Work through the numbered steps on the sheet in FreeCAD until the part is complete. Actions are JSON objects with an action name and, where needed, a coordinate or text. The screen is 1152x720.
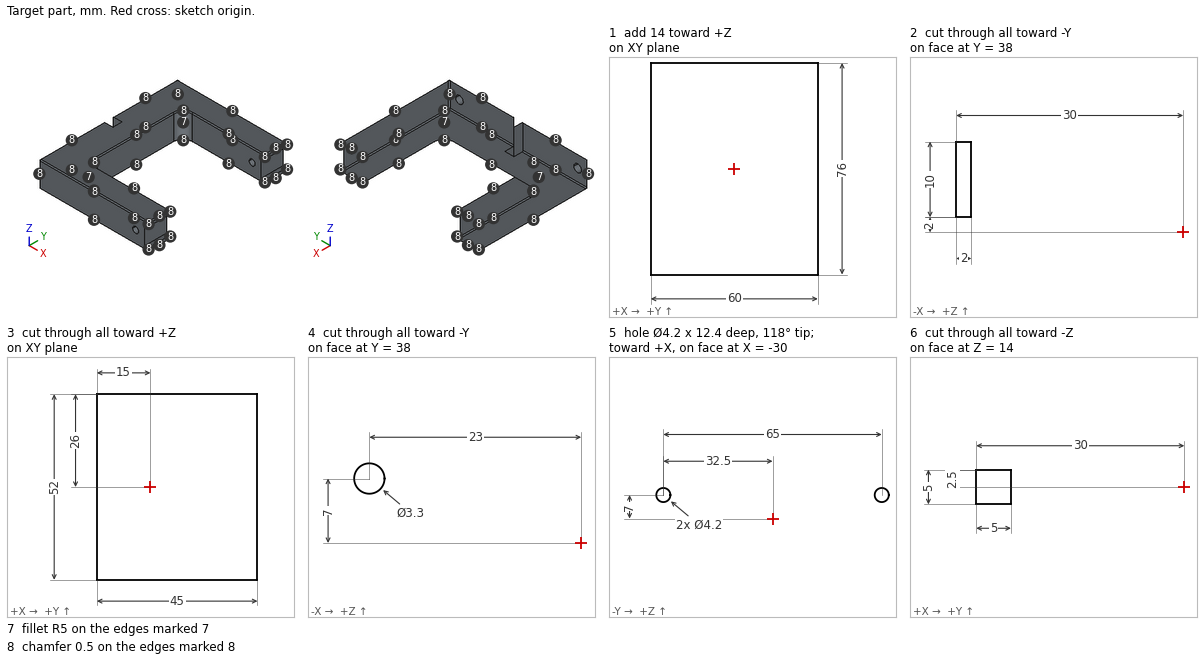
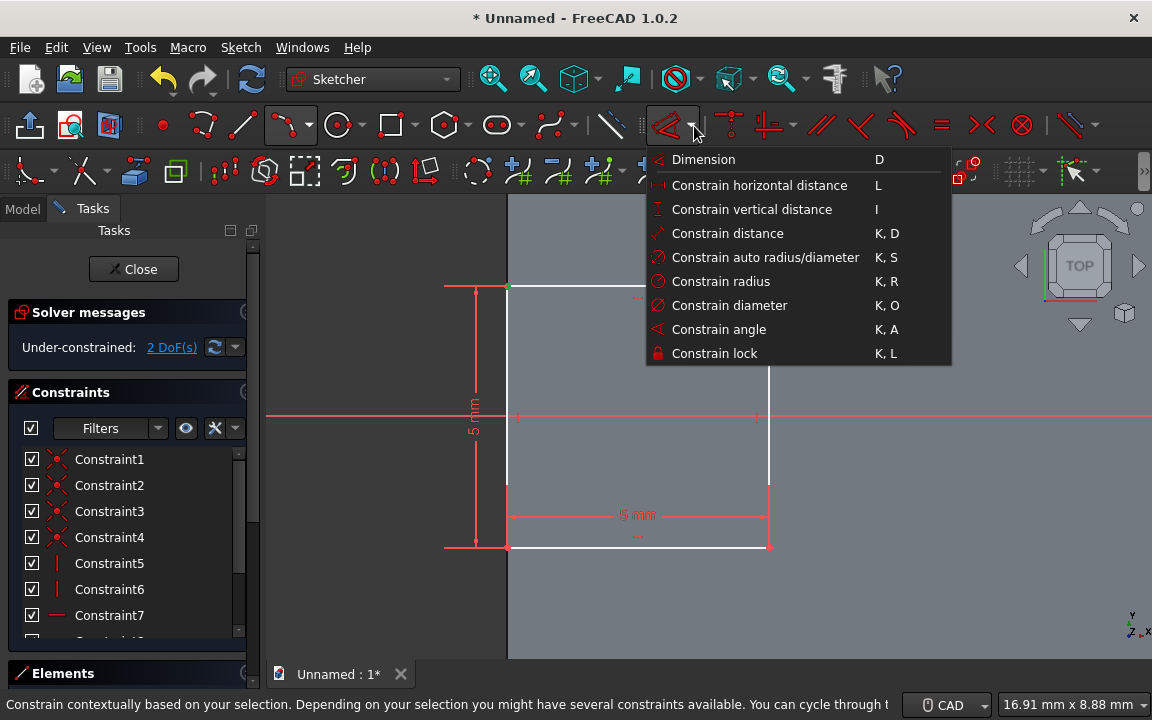
{"action": "left_click", "coordinate": [799, 185]}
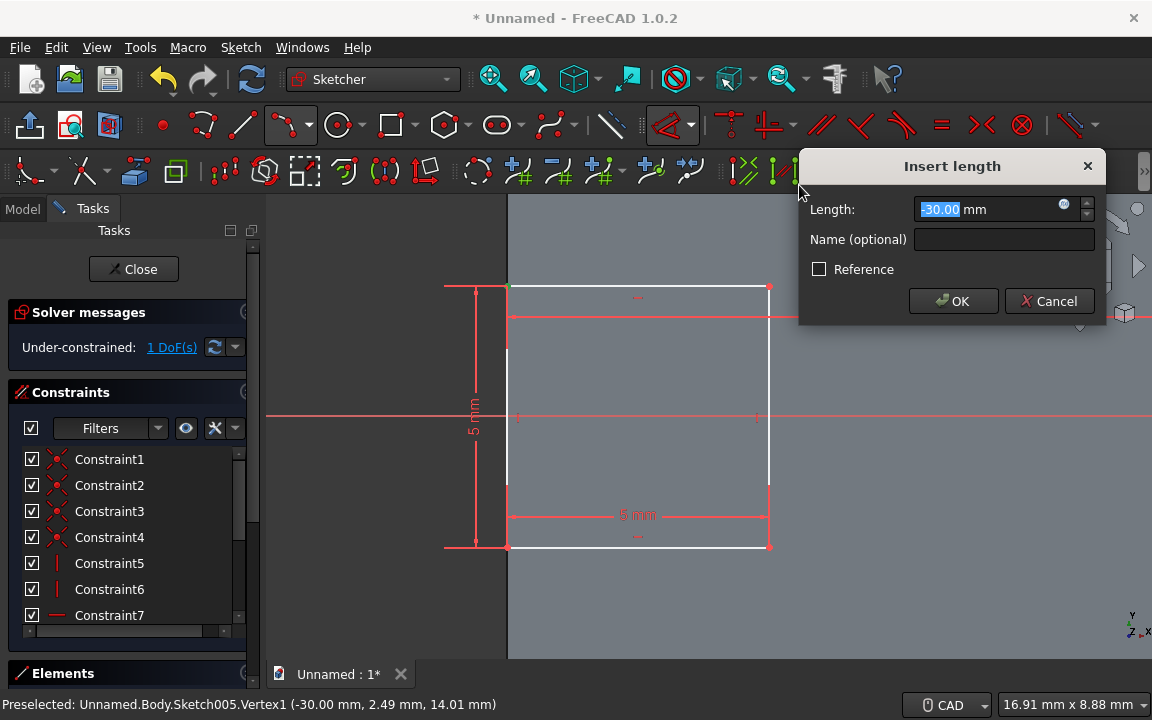
{"action": "type", "text": "-30"}
{"action": "key", "text": "Return"}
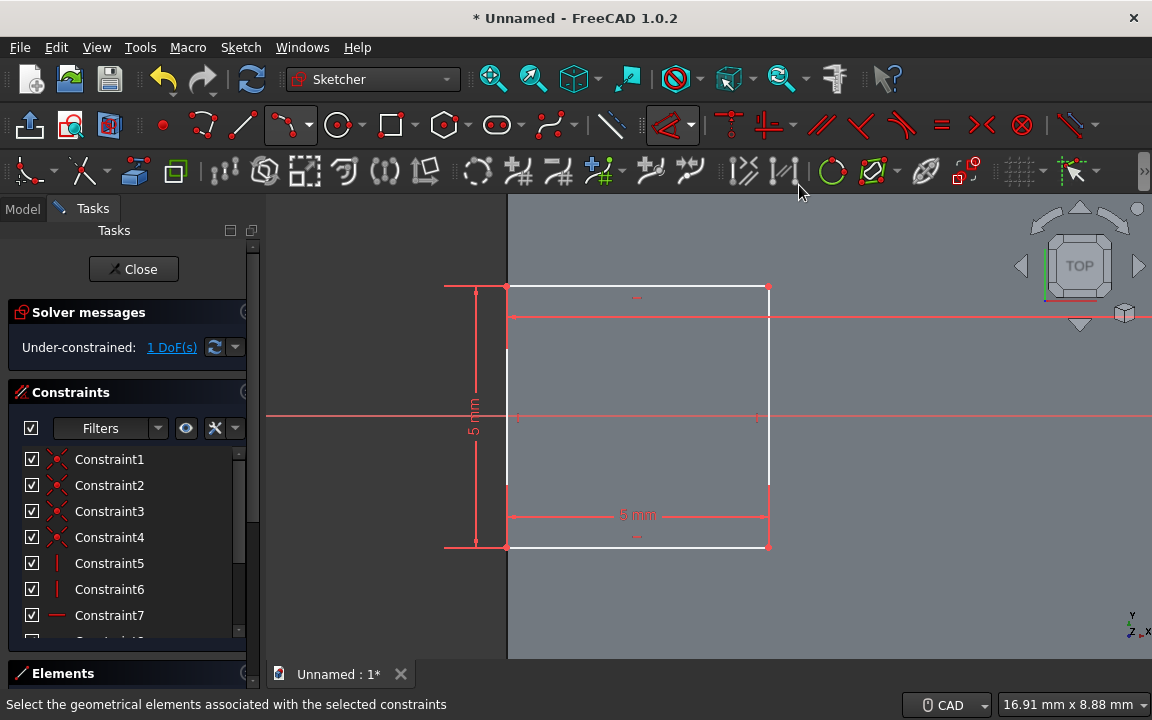
{"action": "left_click", "coordinate": [507, 286]}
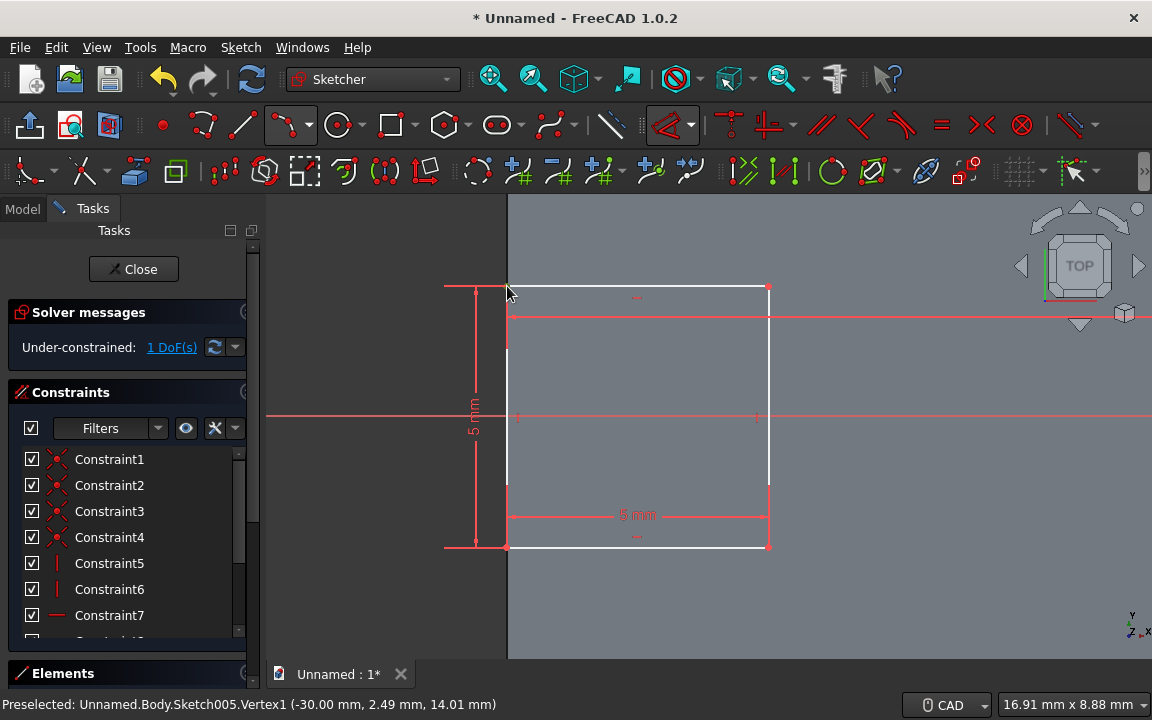
{"action": "key", "text": "i"}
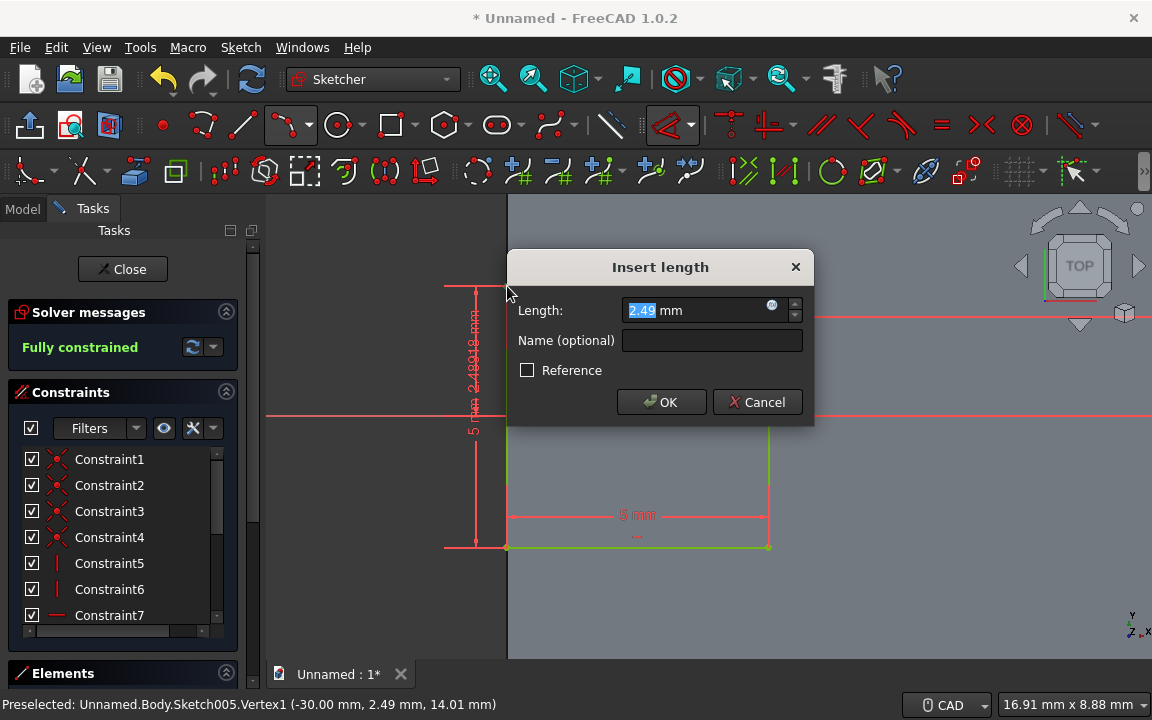
{"action": "type", "text": "2.5"}
{"action": "key", "text": "Return"}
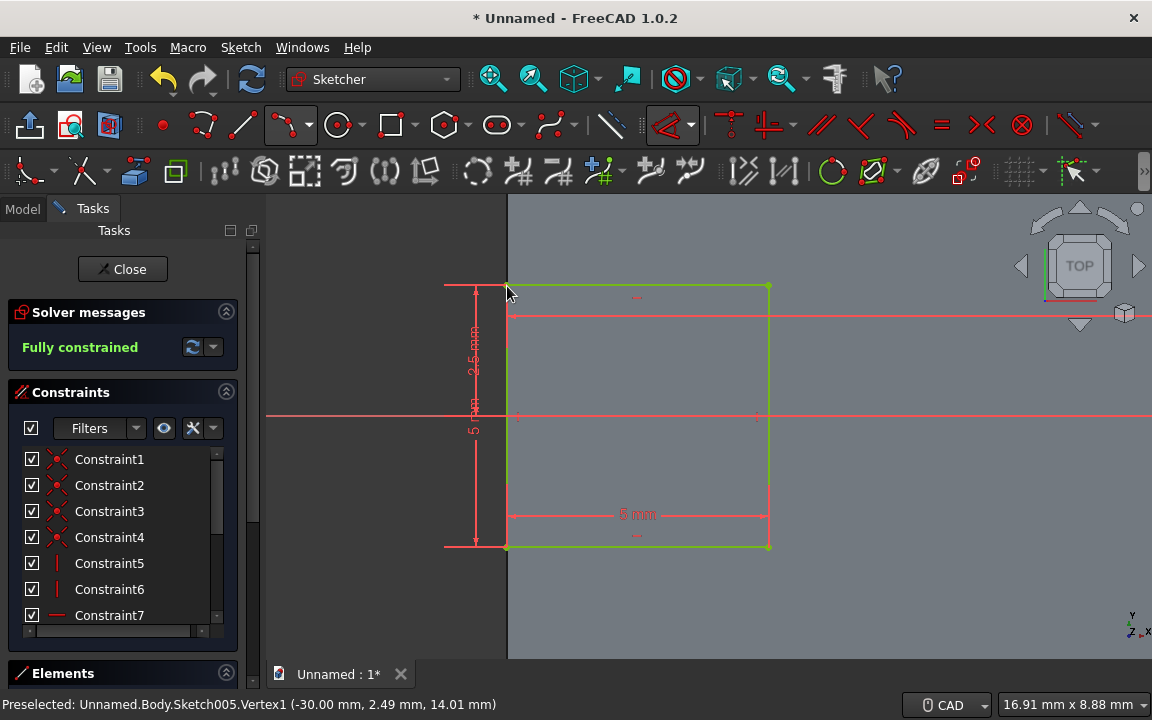
{"action": "left_click", "coordinate": [123, 269]}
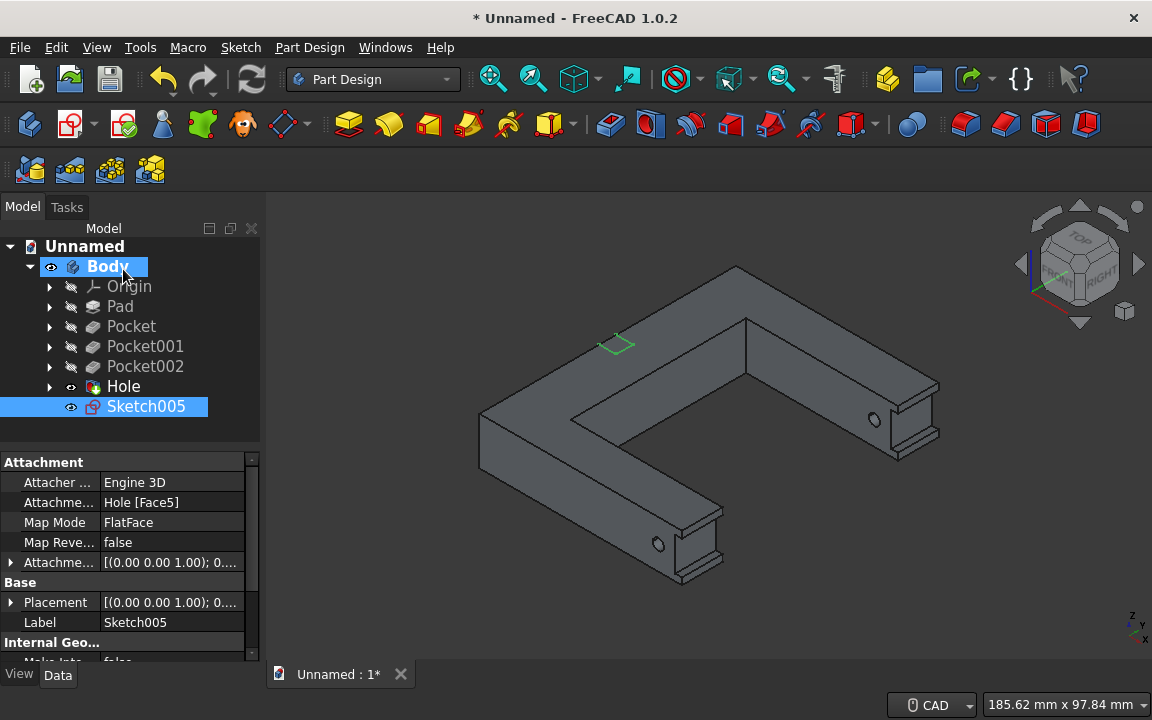
{"action": "left_click", "coordinate": [612, 124]}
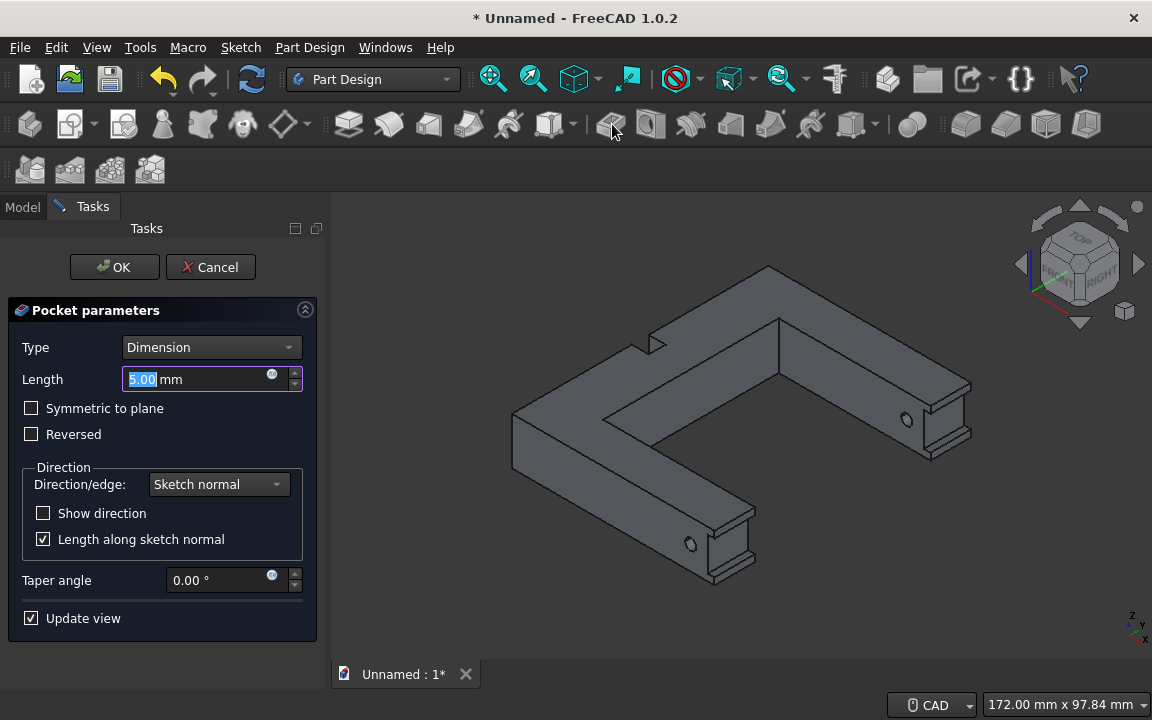
{"action": "left_click", "coordinate": [212, 348]}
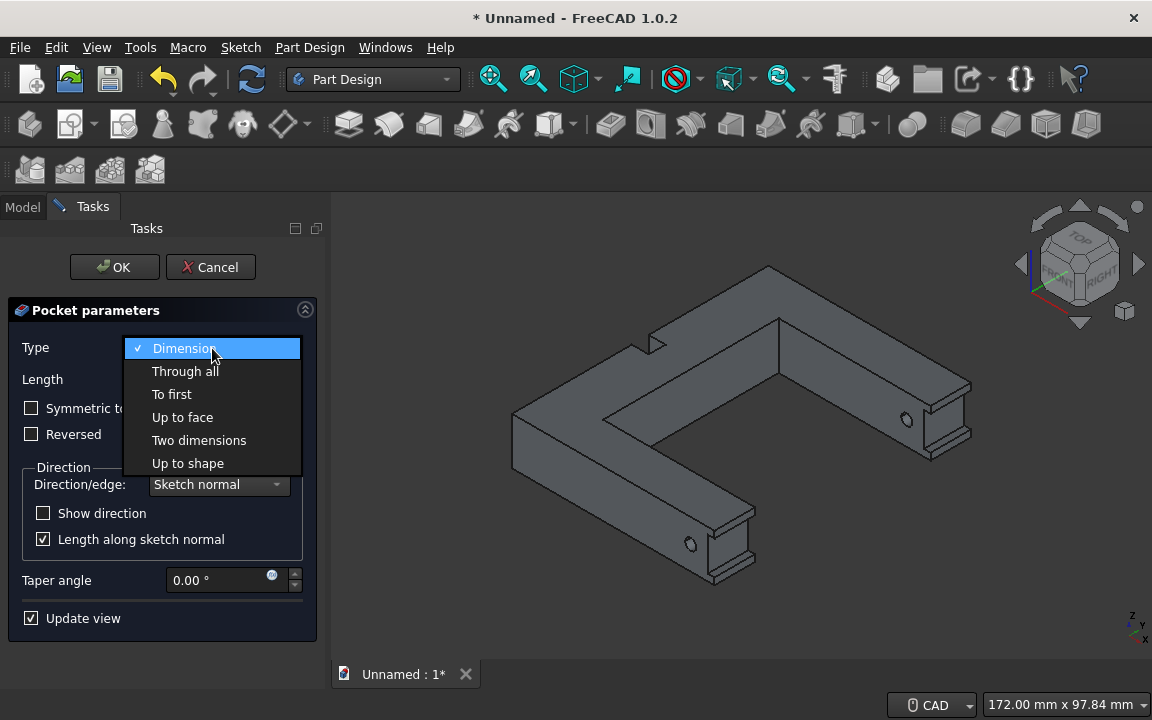
{"action": "left_click", "coordinate": [212, 372]}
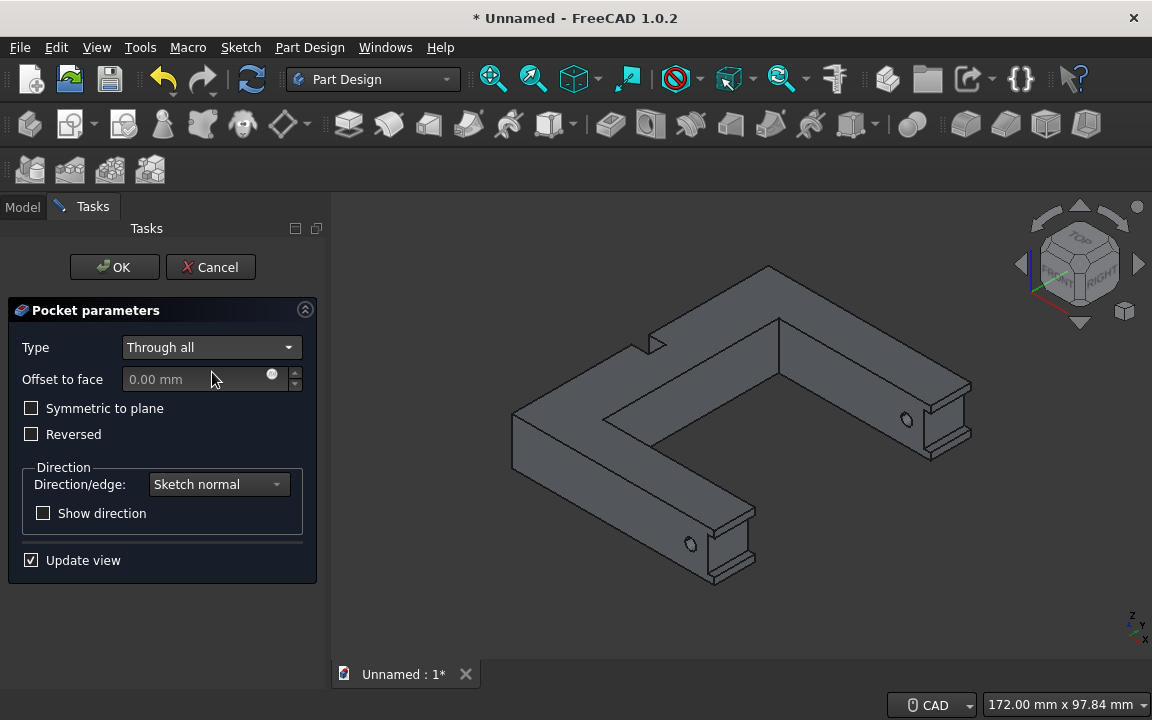
{"action": "left_click", "coordinate": [115, 267]}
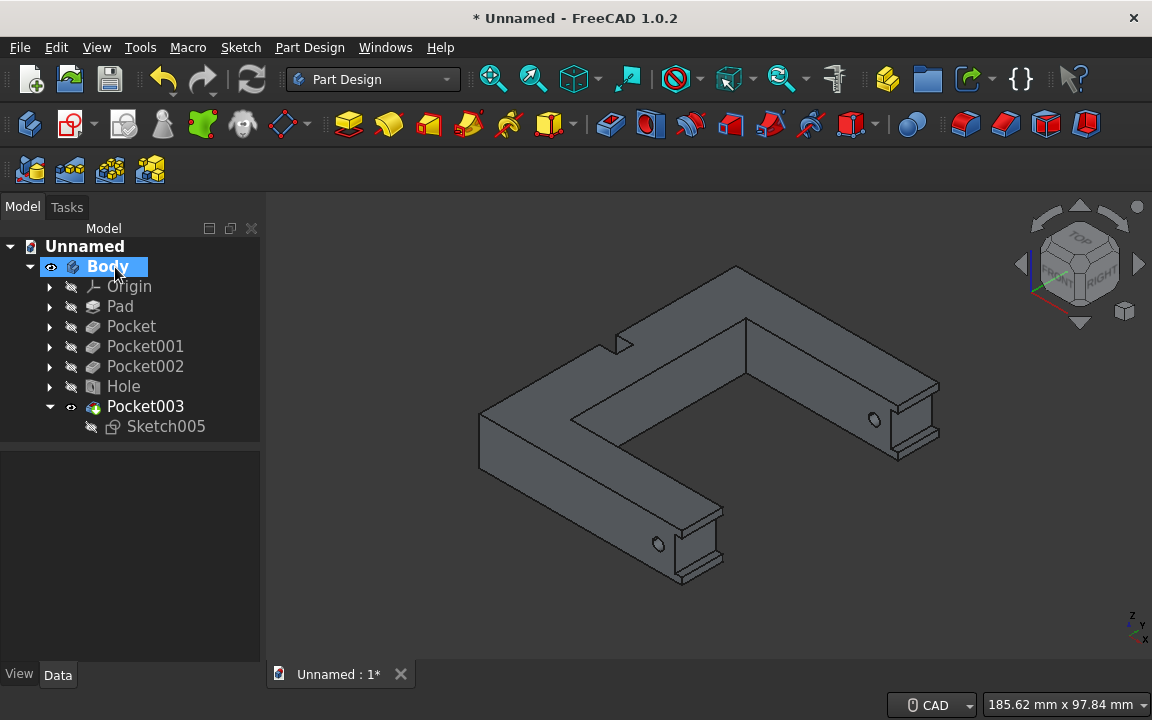
{"action": "key", "text": "2"}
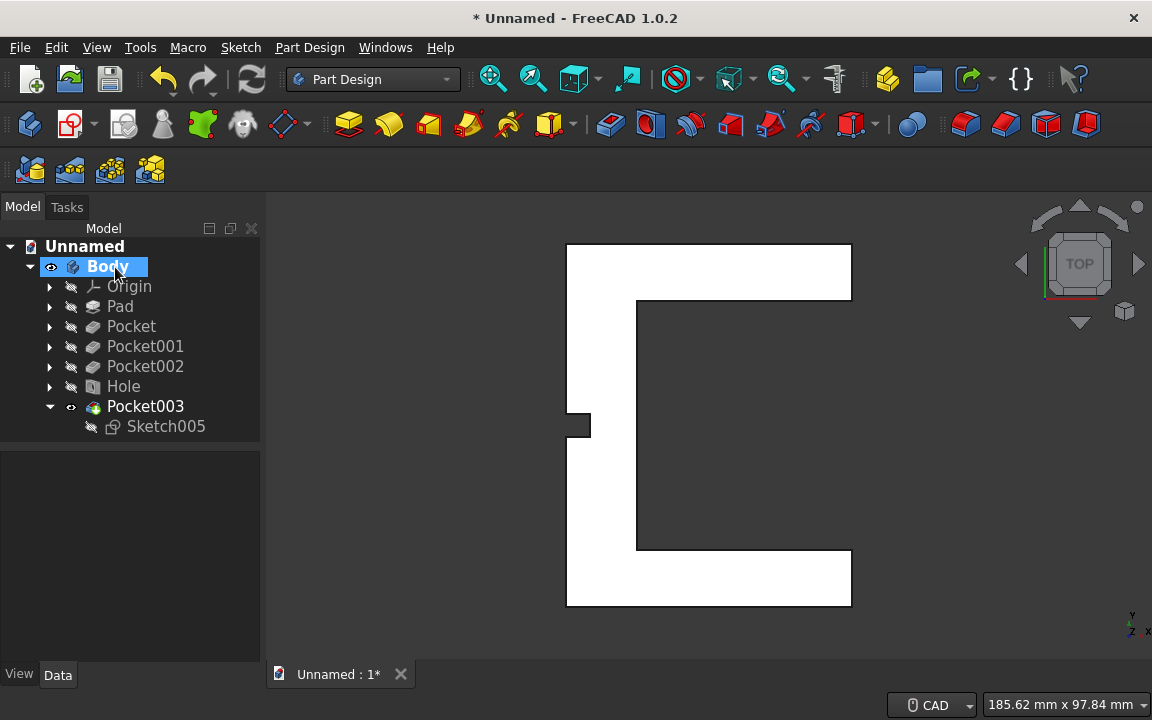
{"action": "key", "text": "0"}